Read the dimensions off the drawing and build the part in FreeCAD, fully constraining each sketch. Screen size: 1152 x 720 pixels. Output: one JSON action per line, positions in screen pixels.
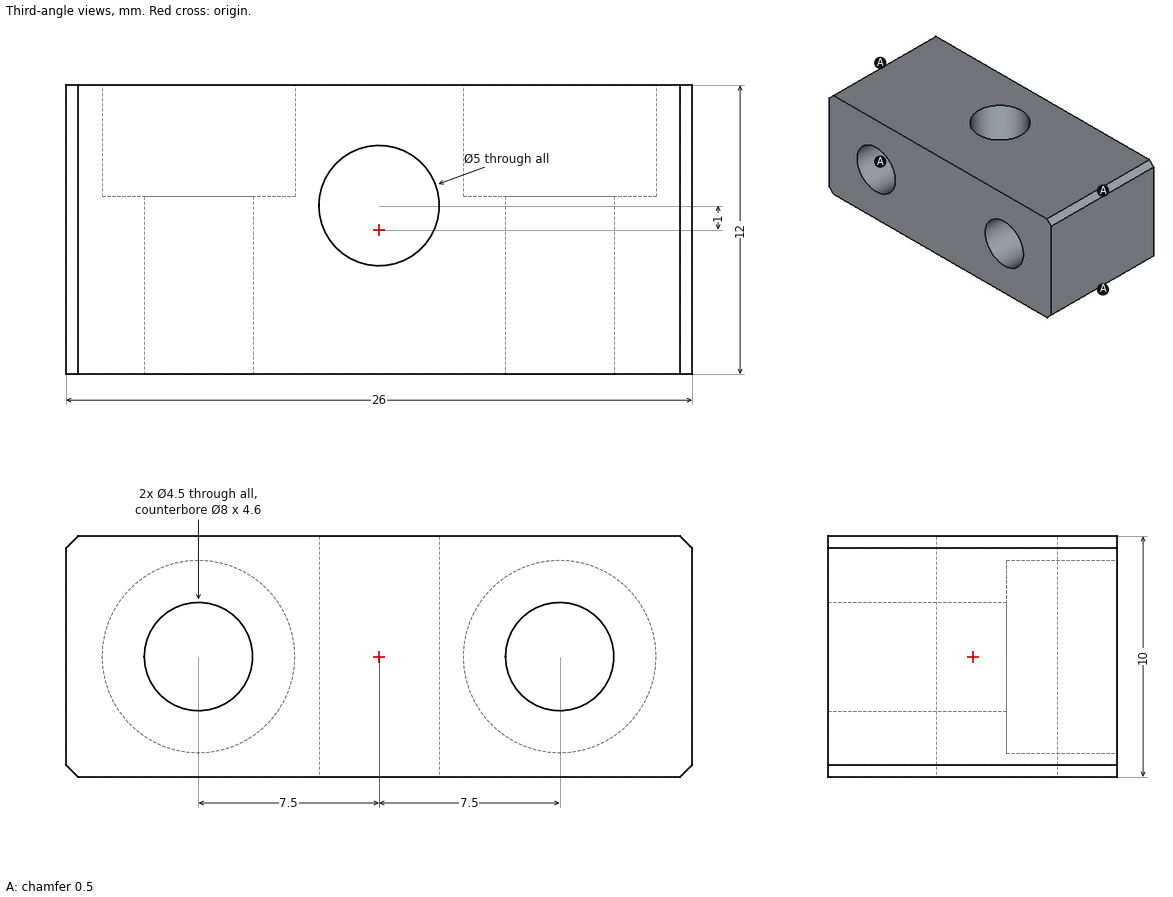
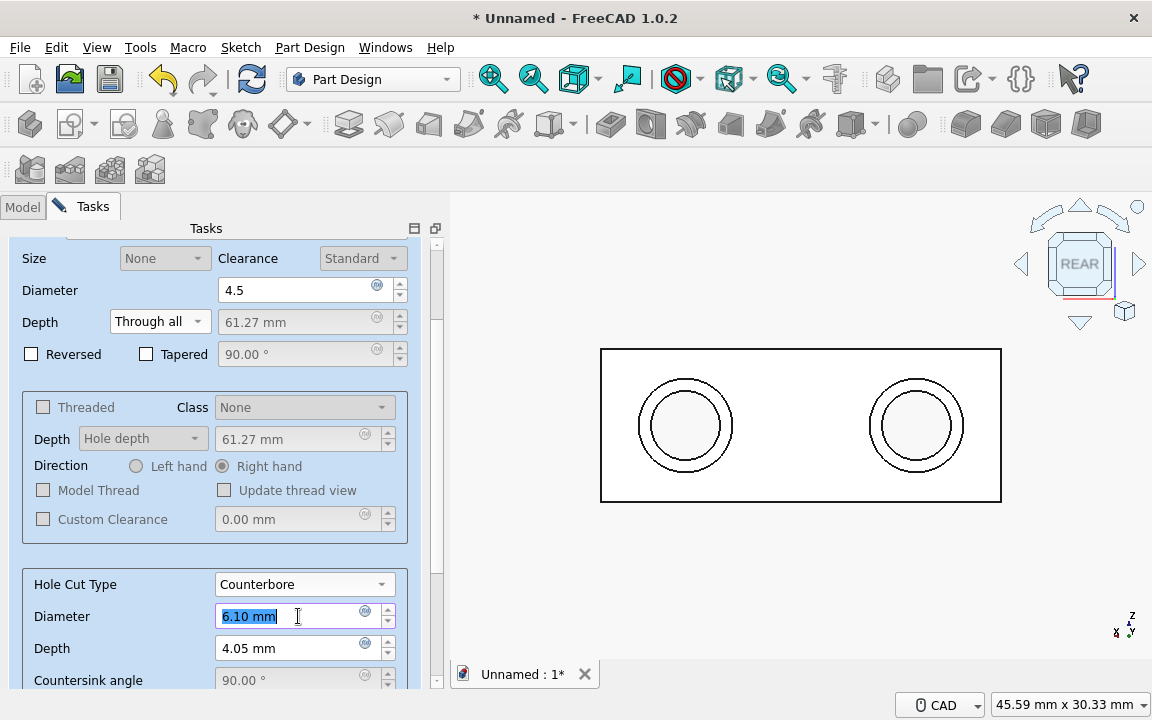
{"action": "type", "text": "8"}
{"action": "key", "text": "Tab"}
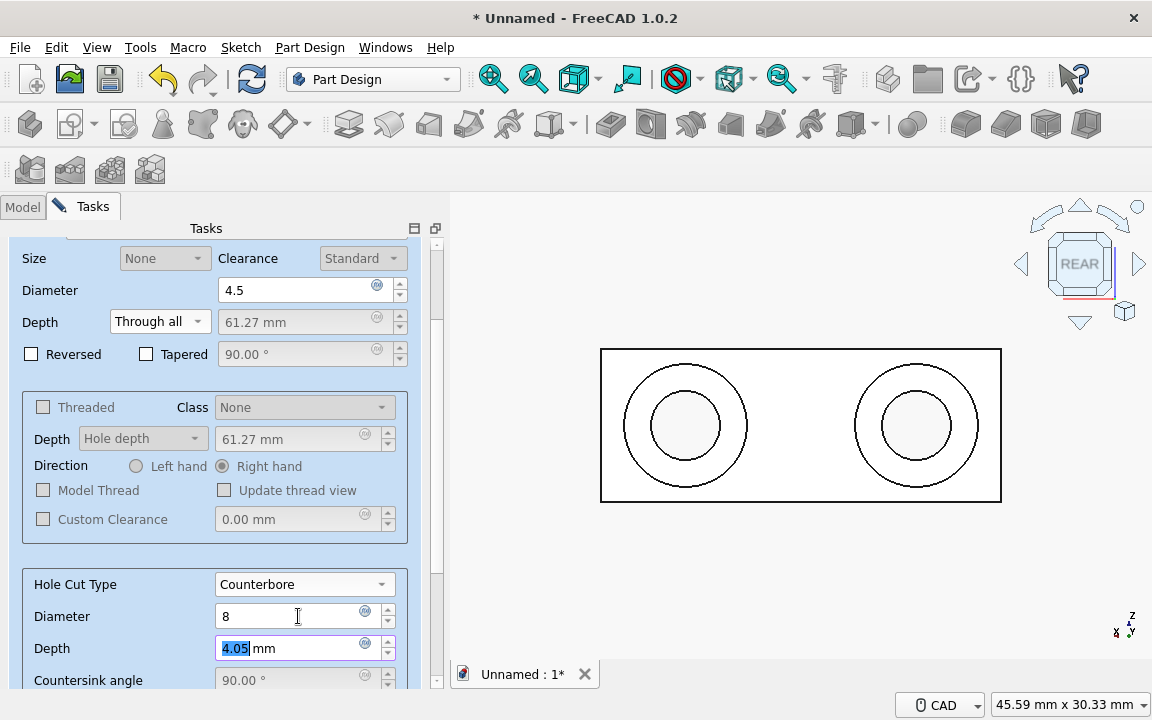
{"action": "type", "text": "4.6"}
{"action": "key", "text": "Tab"}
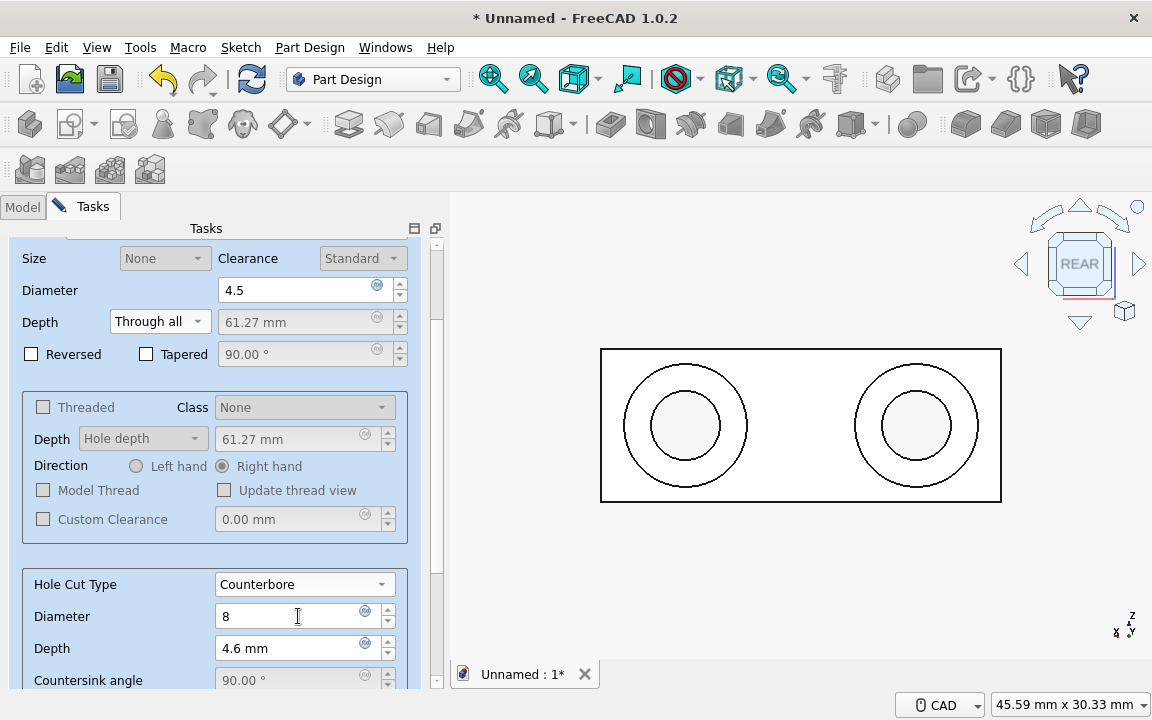
{"action": "scroll", "coordinate": [437, 463], "scroll_direction": "up", "scroll_amount": 3}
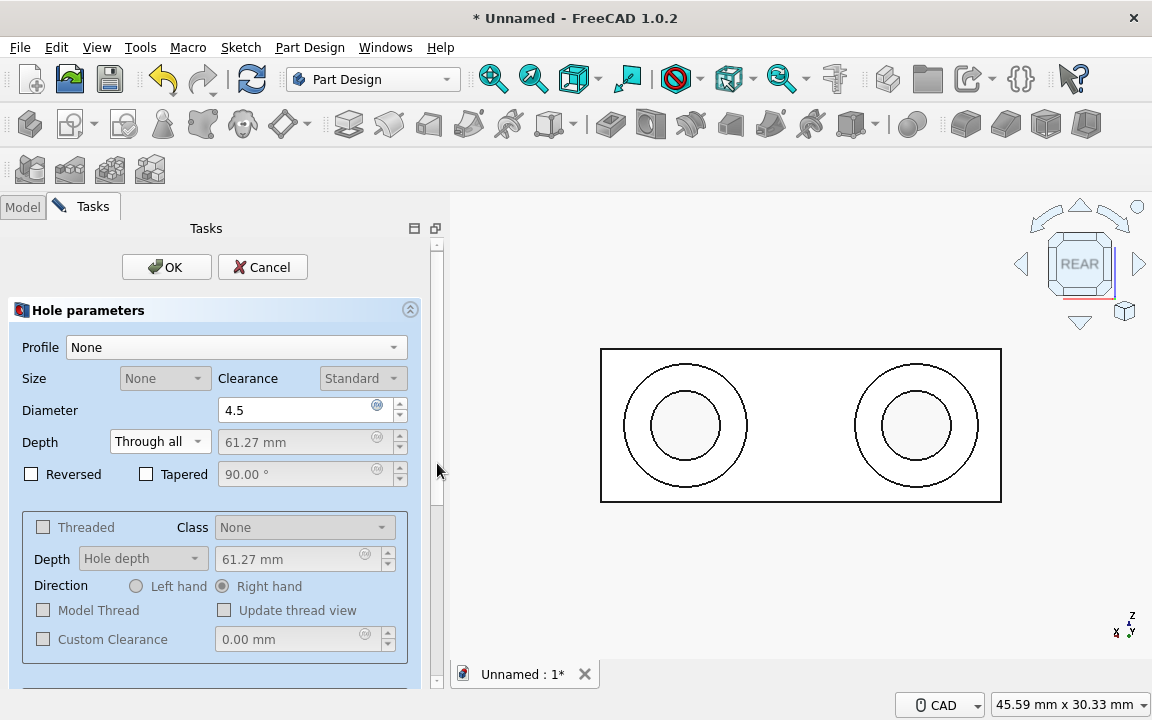
{"action": "left_click", "coordinate": [167, 267]}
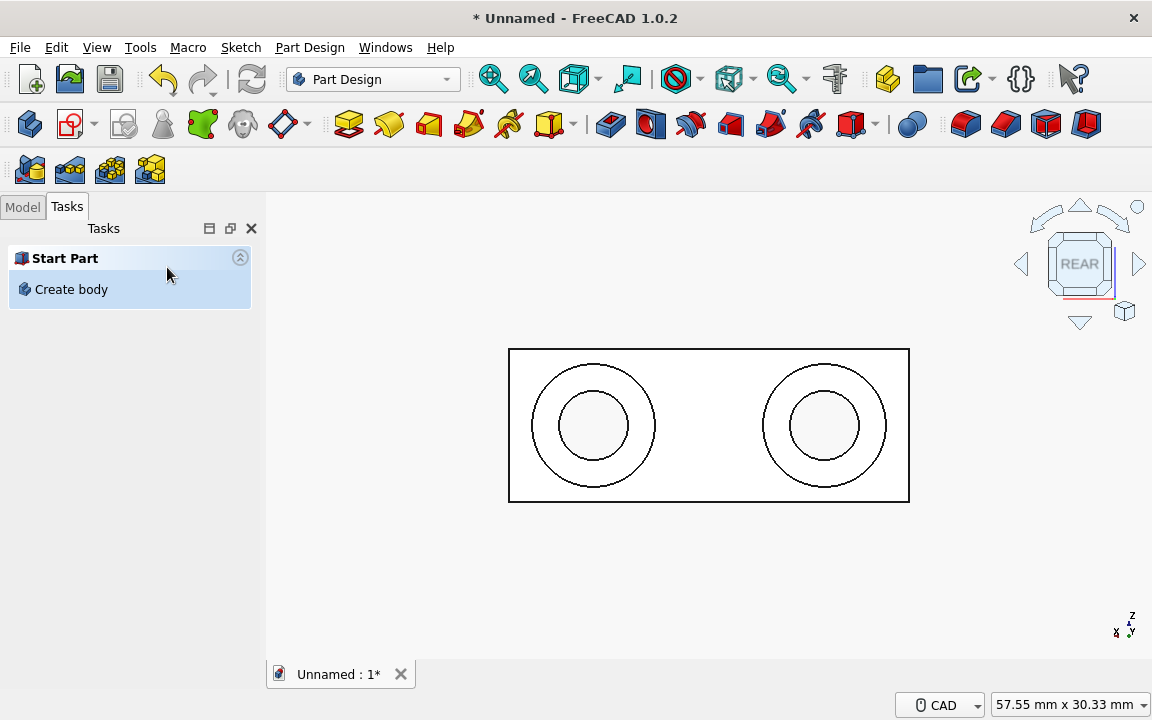
{"action": "key", "text": "0"}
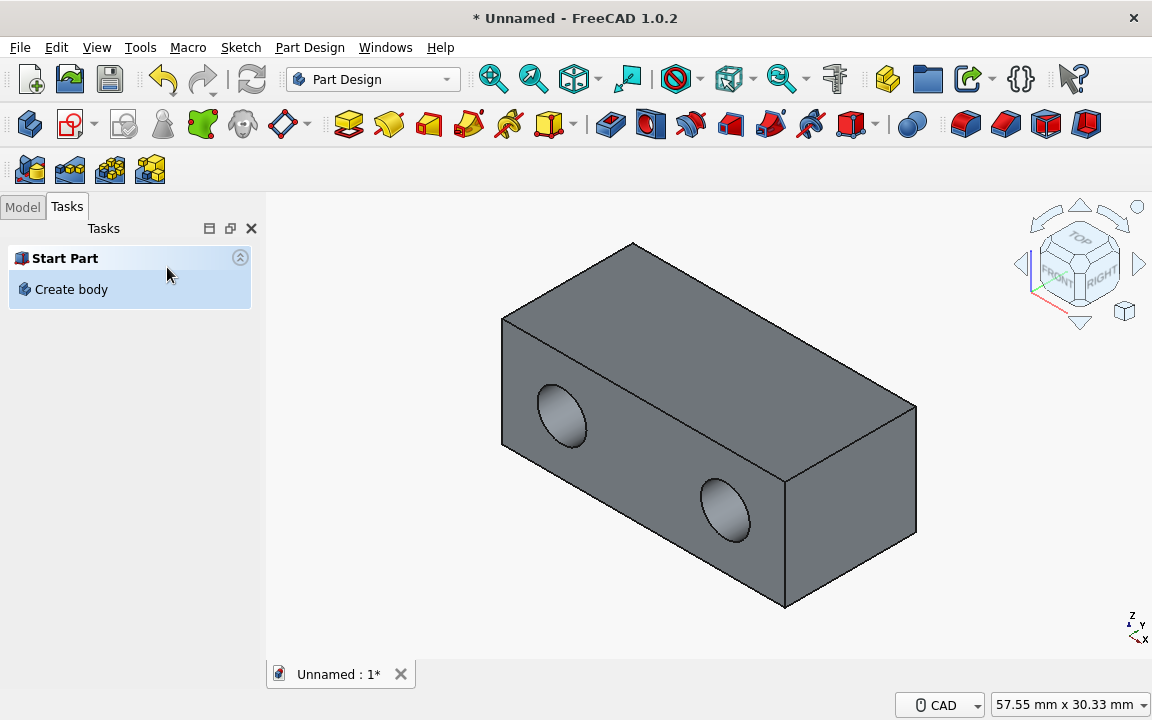
{"action": "left_click", "coordinate": [749, 385]}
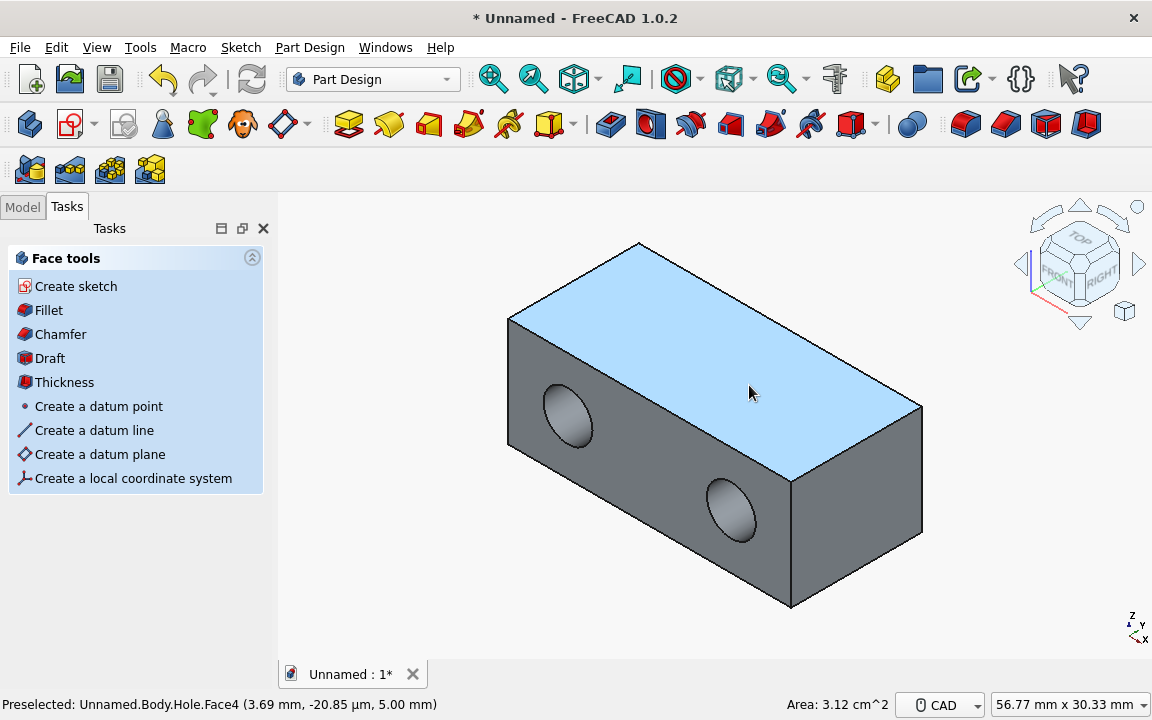
{"action": "left_click", "coordinate": [70, 124]}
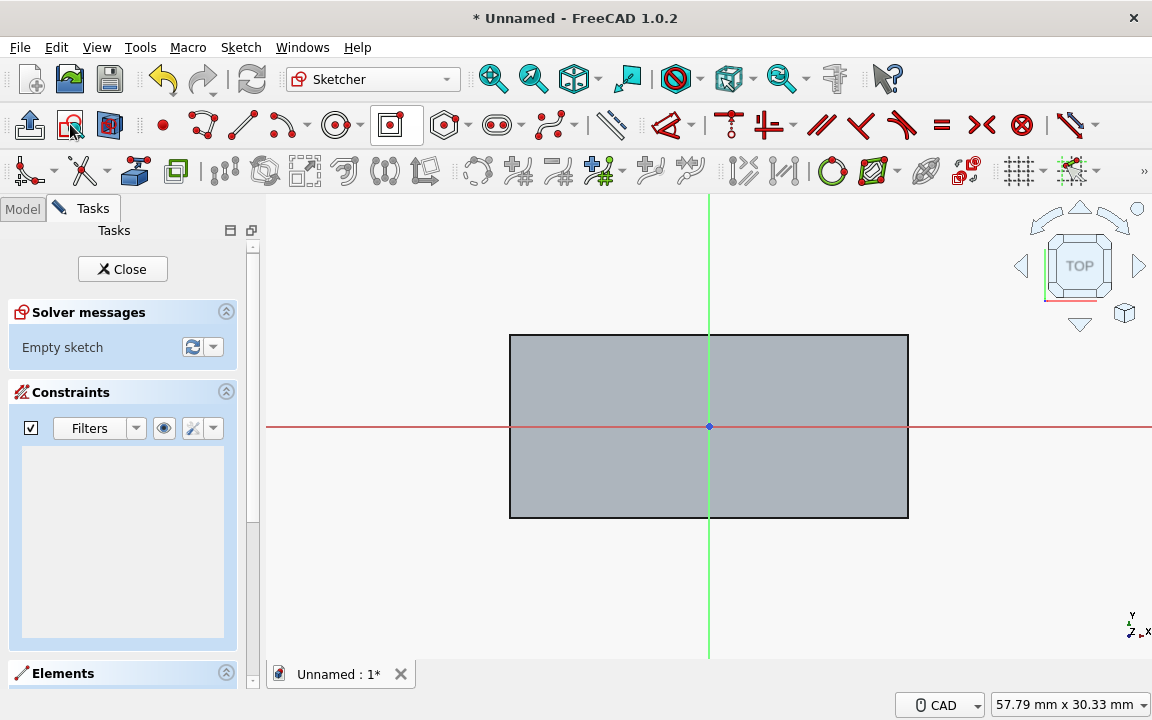
{"action": "scroll", "coordinate": [731, 406], "scroll_direction": "up", "scroll_amount": 7}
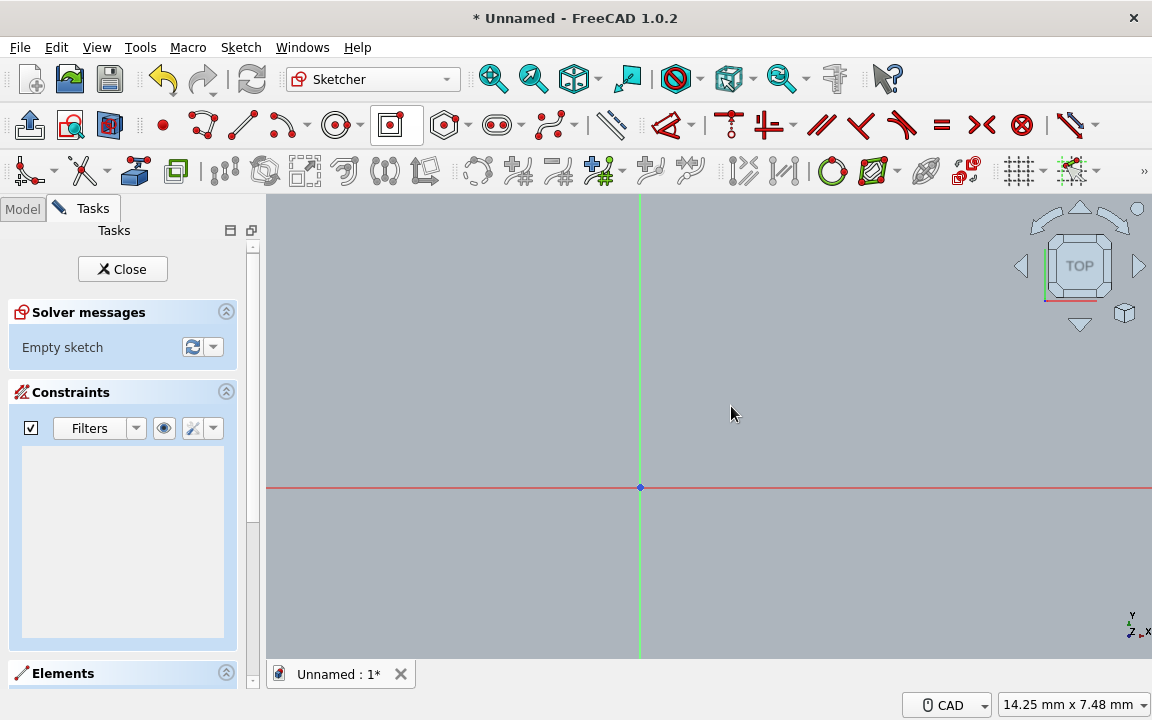
{"action": "key", "text": "g c"}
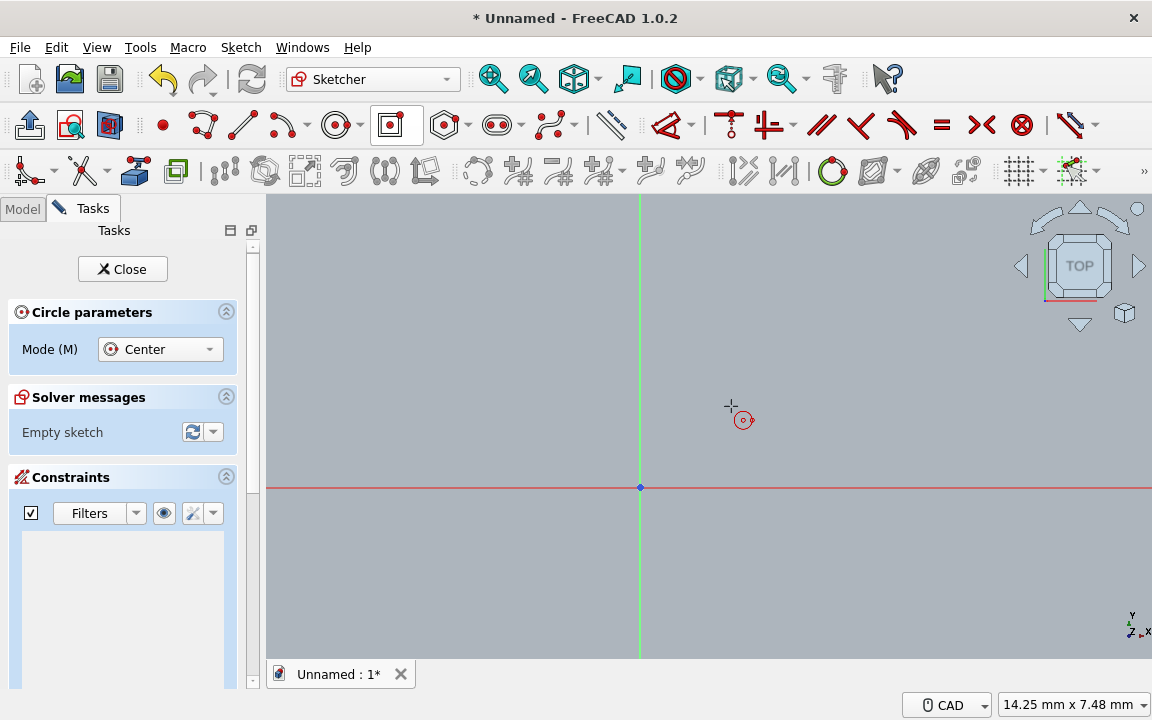
{"action": "left_click", "coordinate": [640, 426]}
{"action": "left_click", "coordinate": [750, 316]}
{"action": "key", "text": "Escape"}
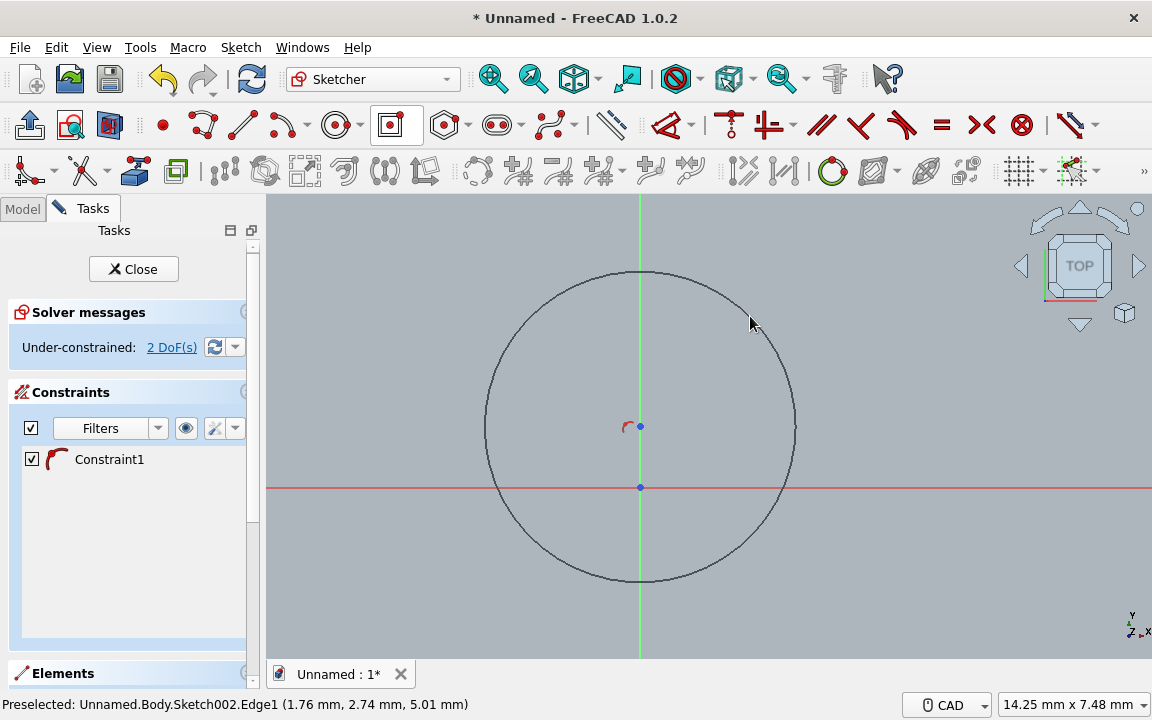
{"action": "left_click", "coordinate": [750, 317]}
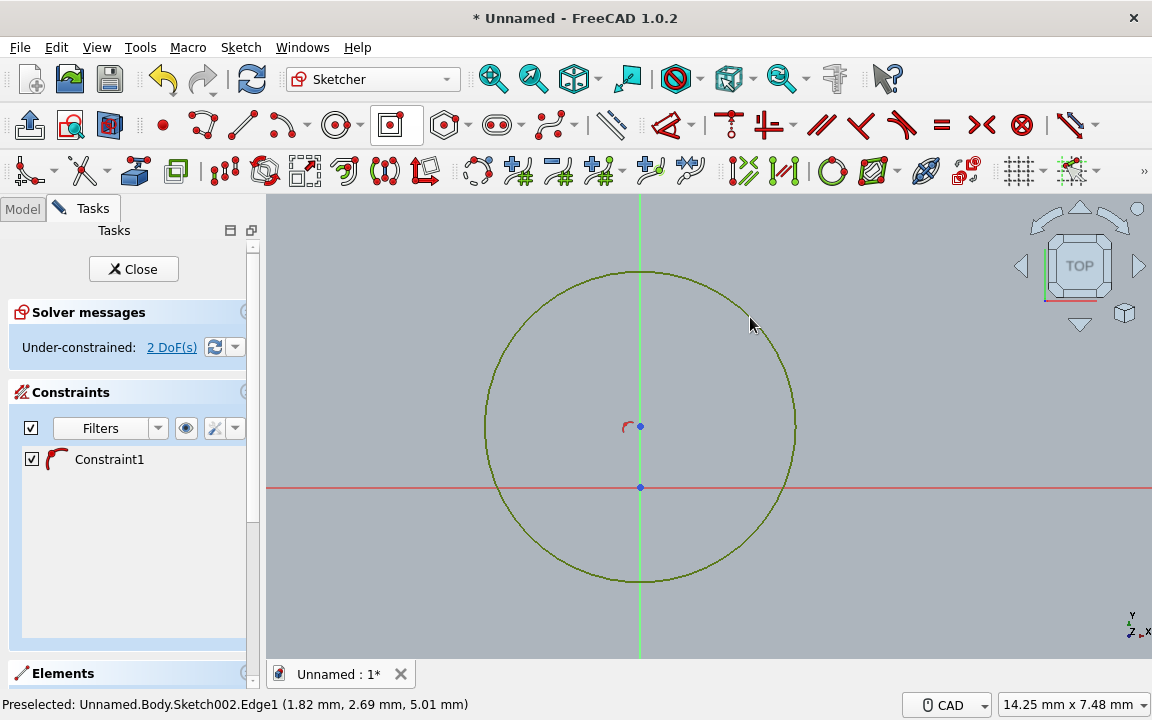
{"action": "key", "text": "k o"}